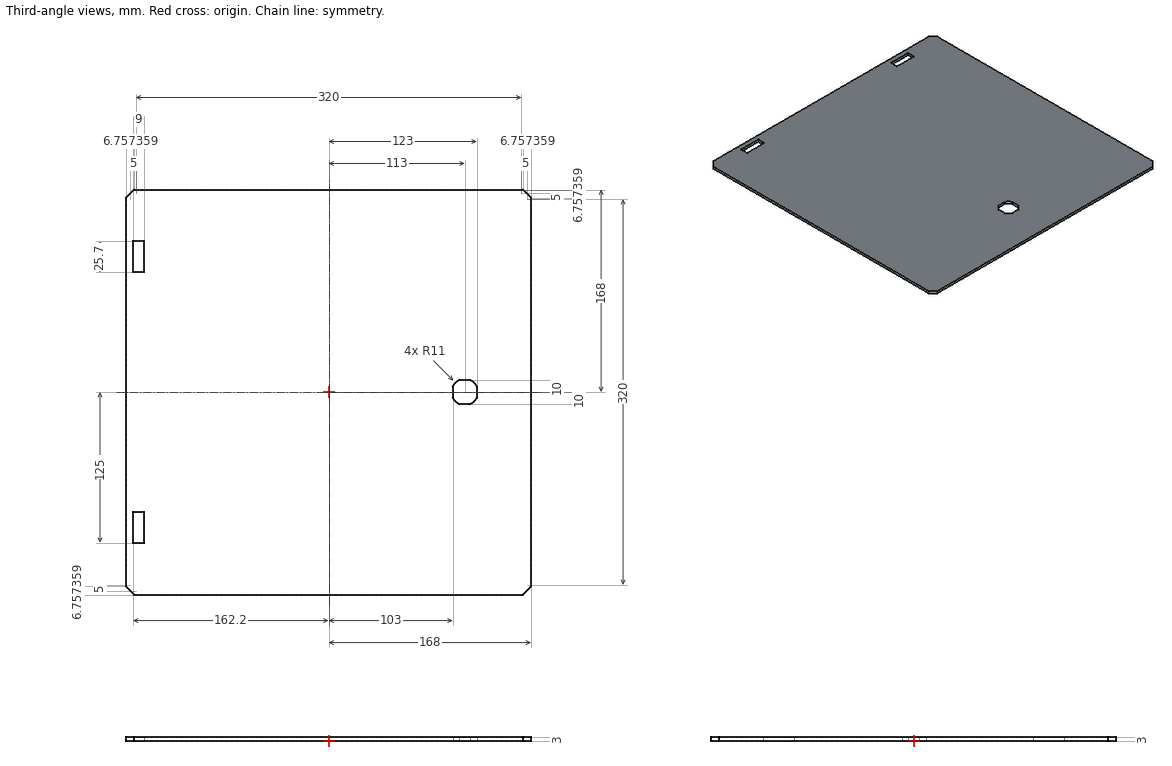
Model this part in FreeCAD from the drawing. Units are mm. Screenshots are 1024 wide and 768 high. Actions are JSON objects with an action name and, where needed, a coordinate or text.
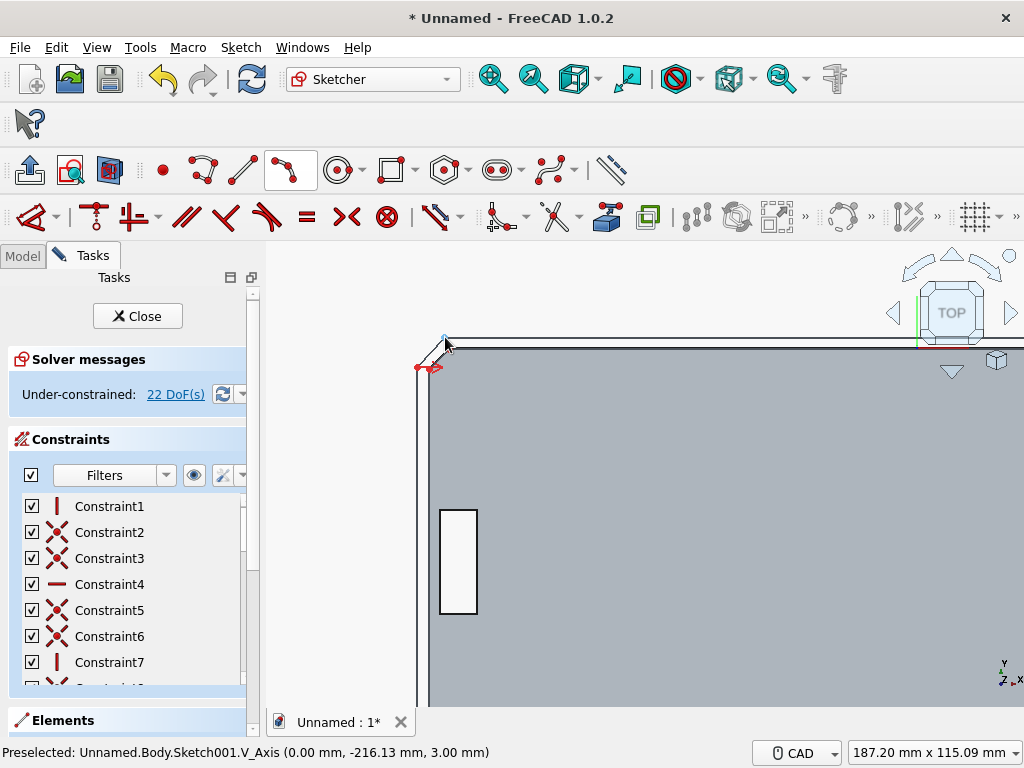
{"action": "left_click", "coordinate": [445, 338]}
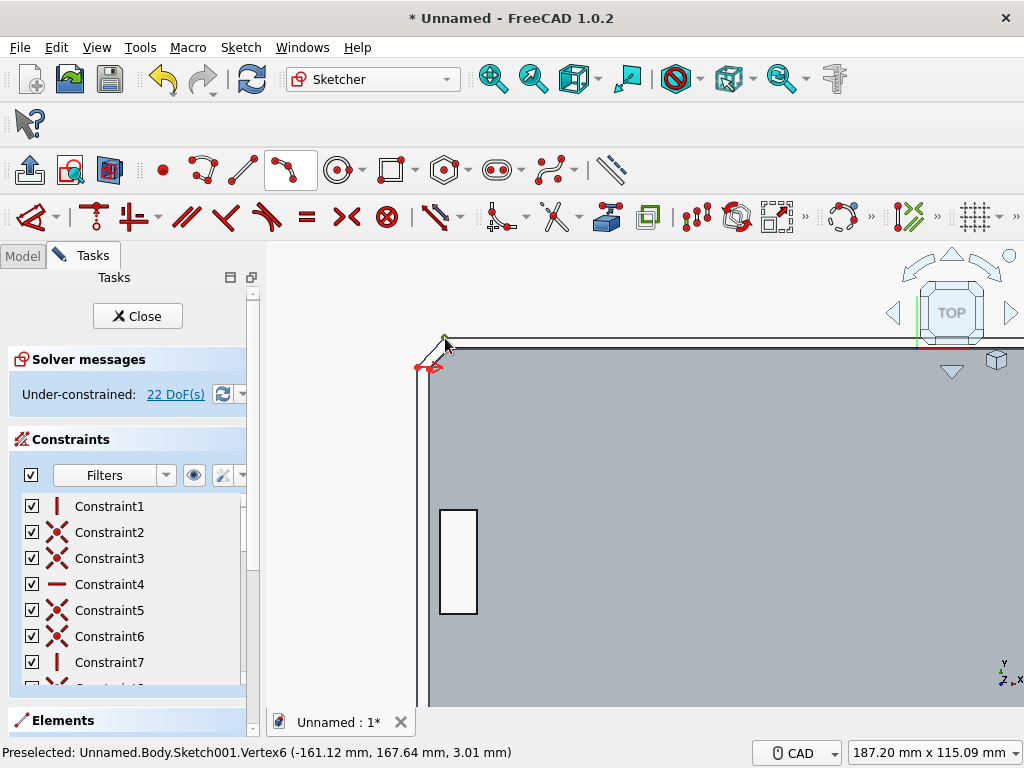
{"action": "scroll", "coordinate": [445, 337], "scroll_direction": "down", "scroll_amount": 8}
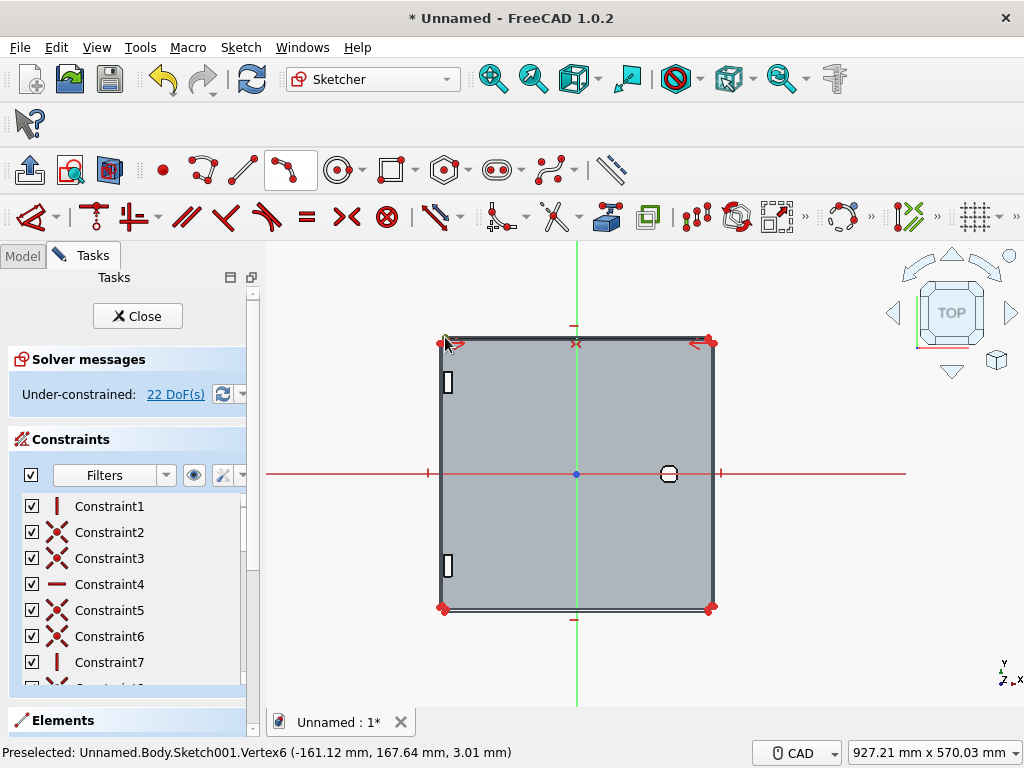
{"action": "scroll", "coordinate": [445, 612], "scroll_direction": "up", "scroll_amount": 7}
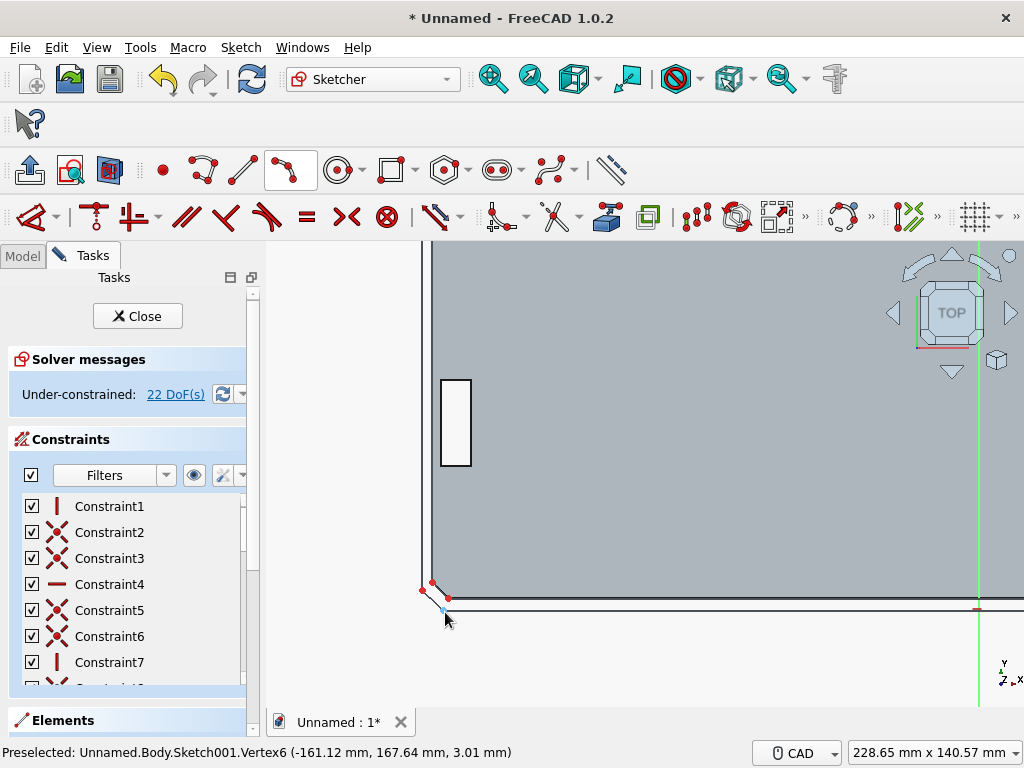
{"action": "left_click", "coordinate": [444, 611]}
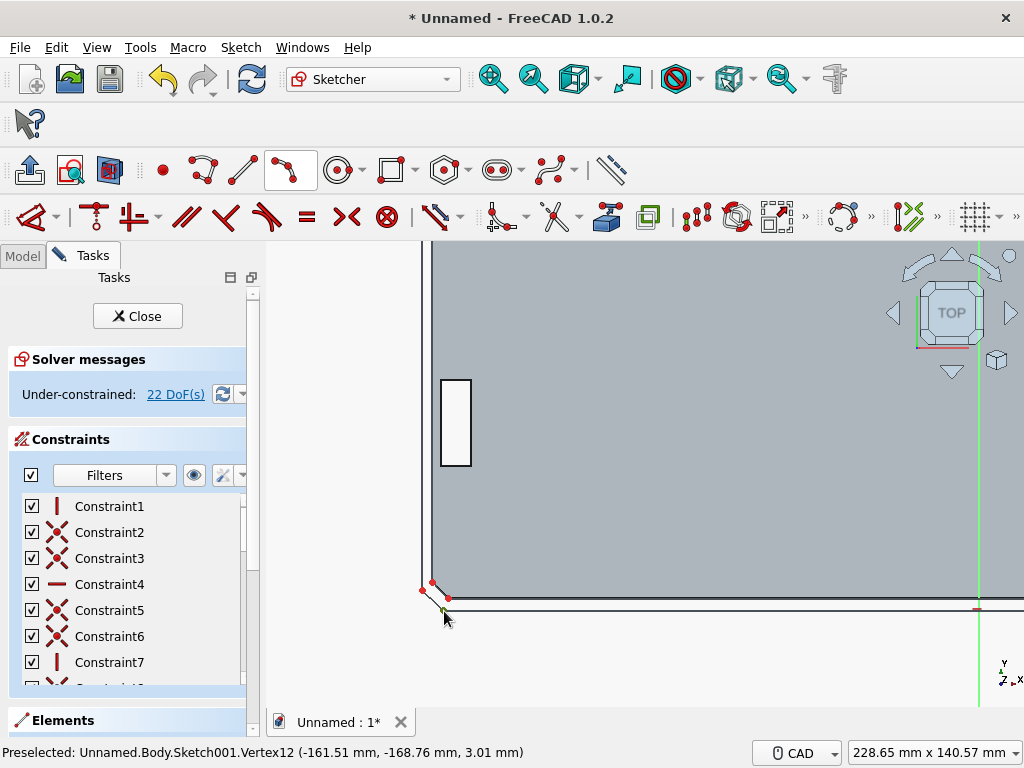
{"action": "scroll", "coordinate": [445, 612], "scroll_direction": "down", "scroll_amount": 7}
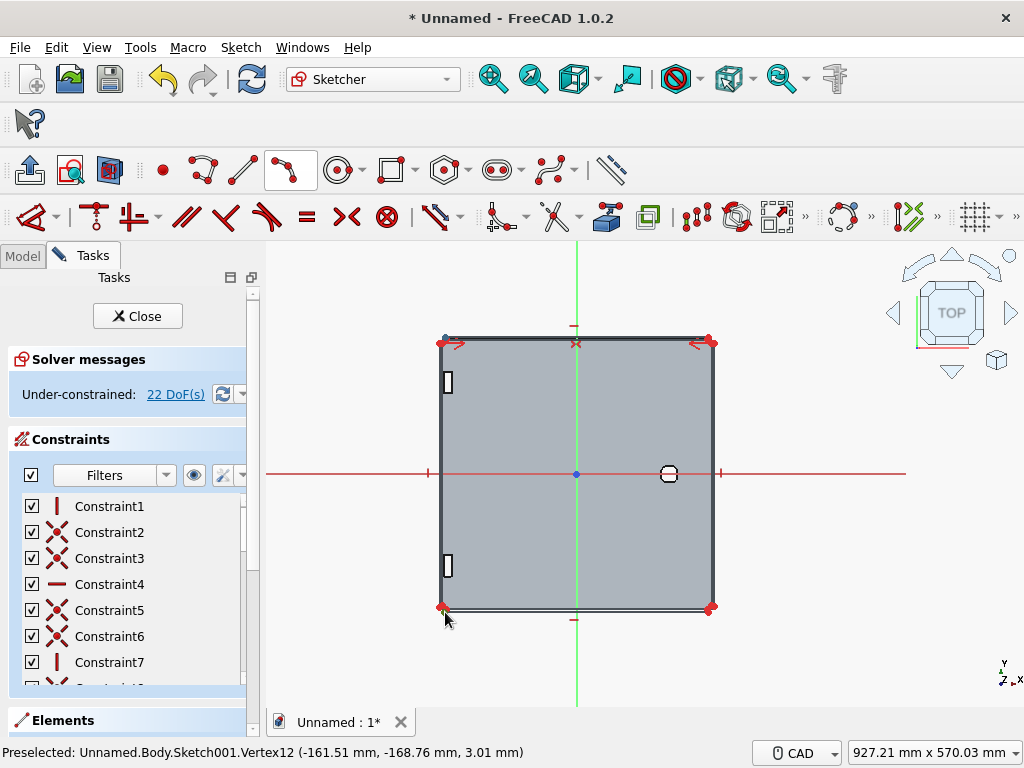
{"action": "left_click", "coordinate": [334, 474]}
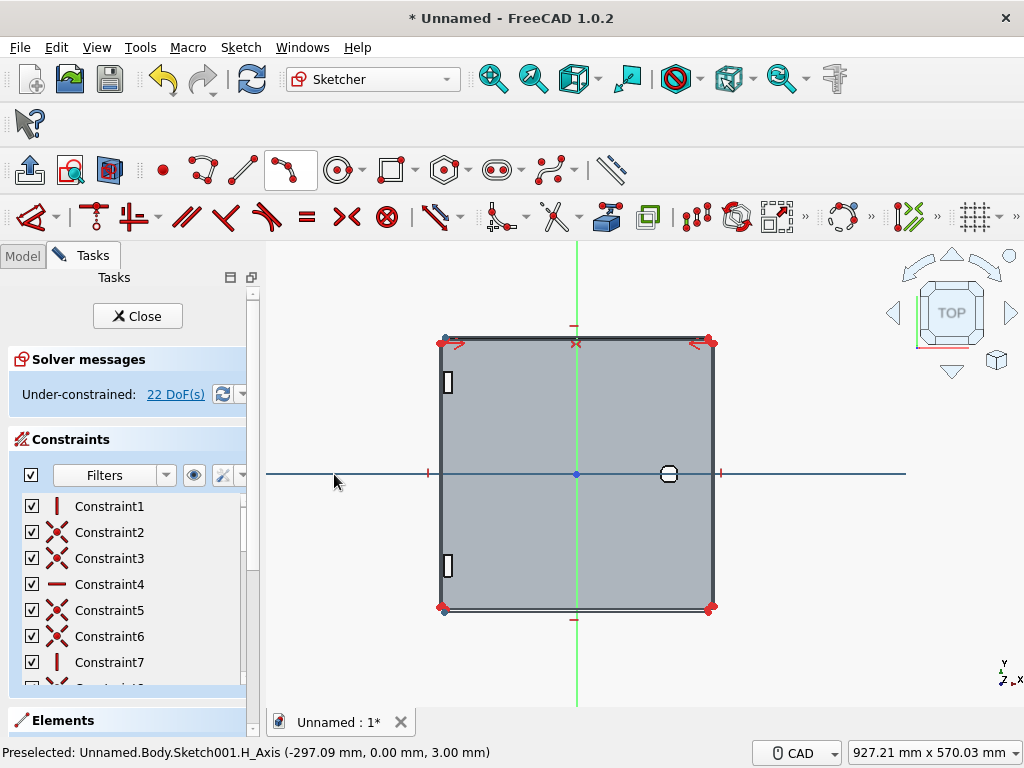
{"action": "left_click", "coordinate": [348, 218]}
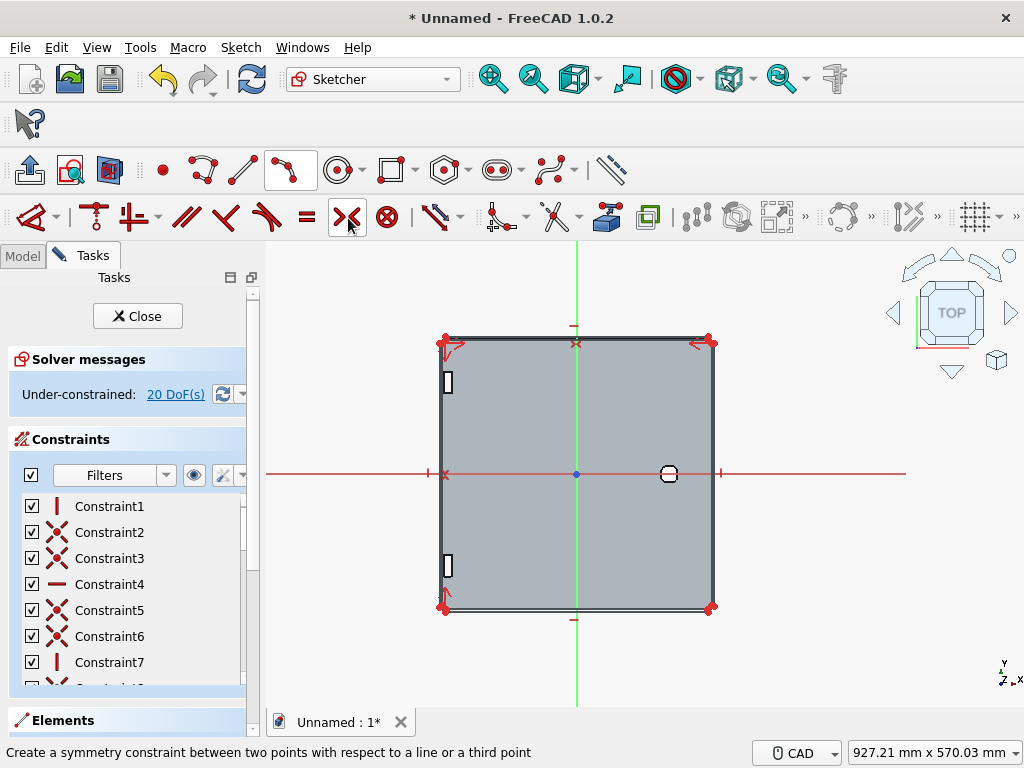
{"action": "scroll", "coordinate": [712, 605], "scroll_direction": "up", "scroll_amount": 8}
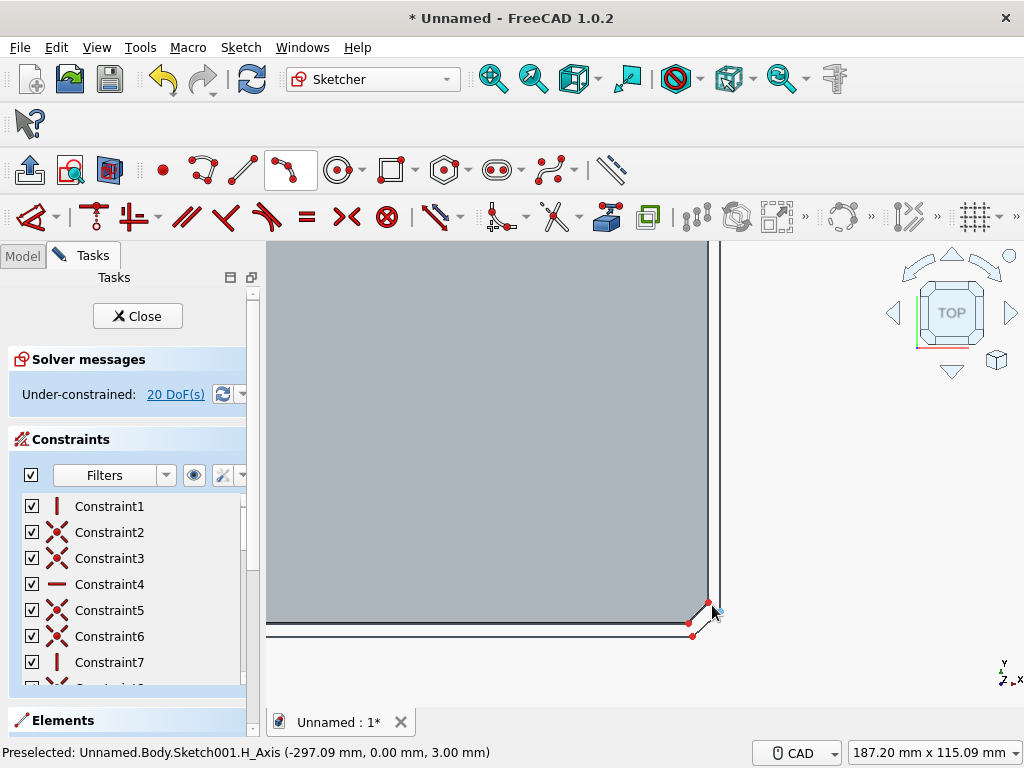
{"action": "left_click", "coordinate": [708, 603]}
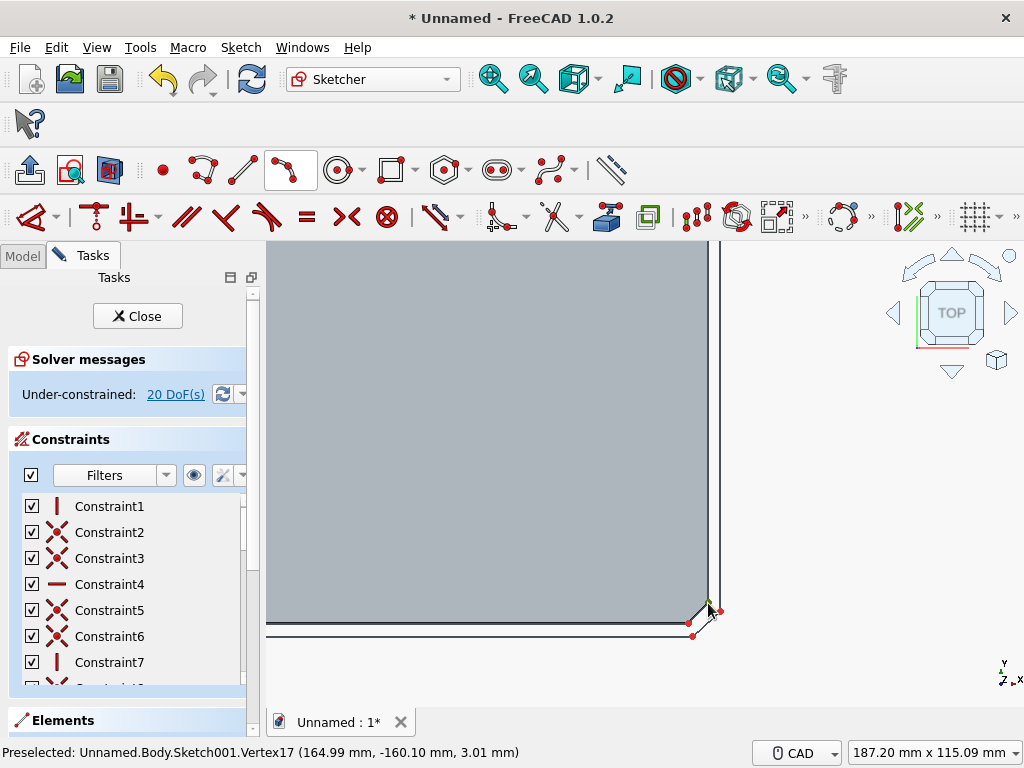
{"action": "scroll", "coordinate": [712, 605], "scroll_direction": "down", "scroll_amount": 8}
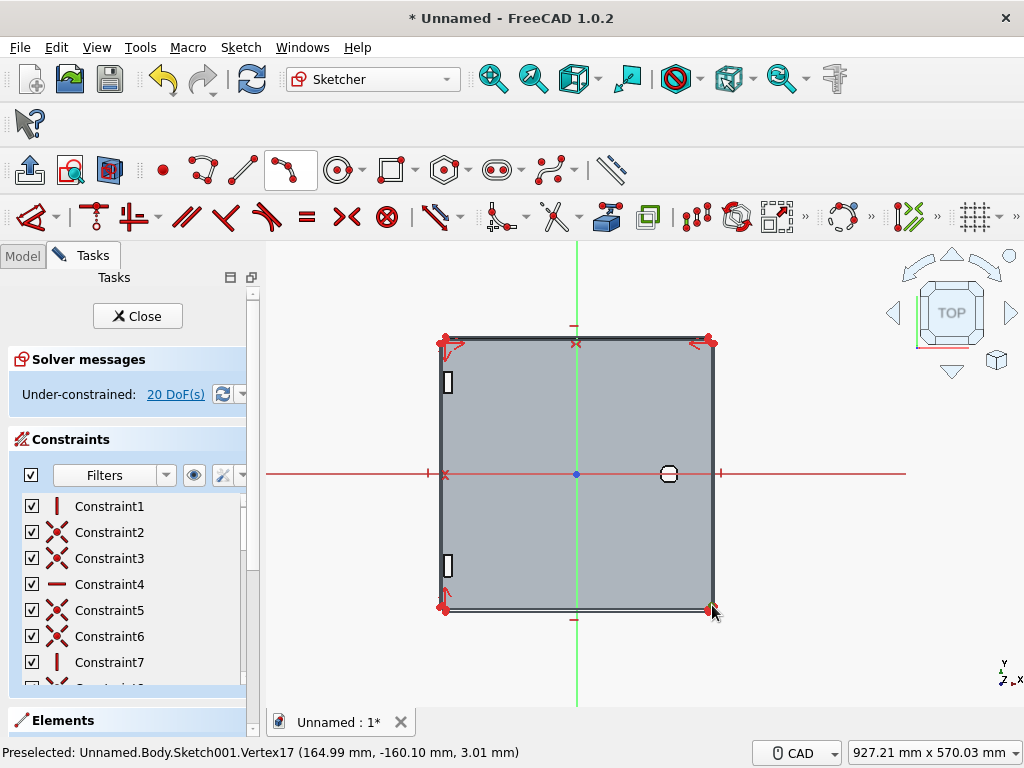
{"action": "scroll", "coordinate": [442, 605], "scroll_direction": "up", "scroll_amount": 7}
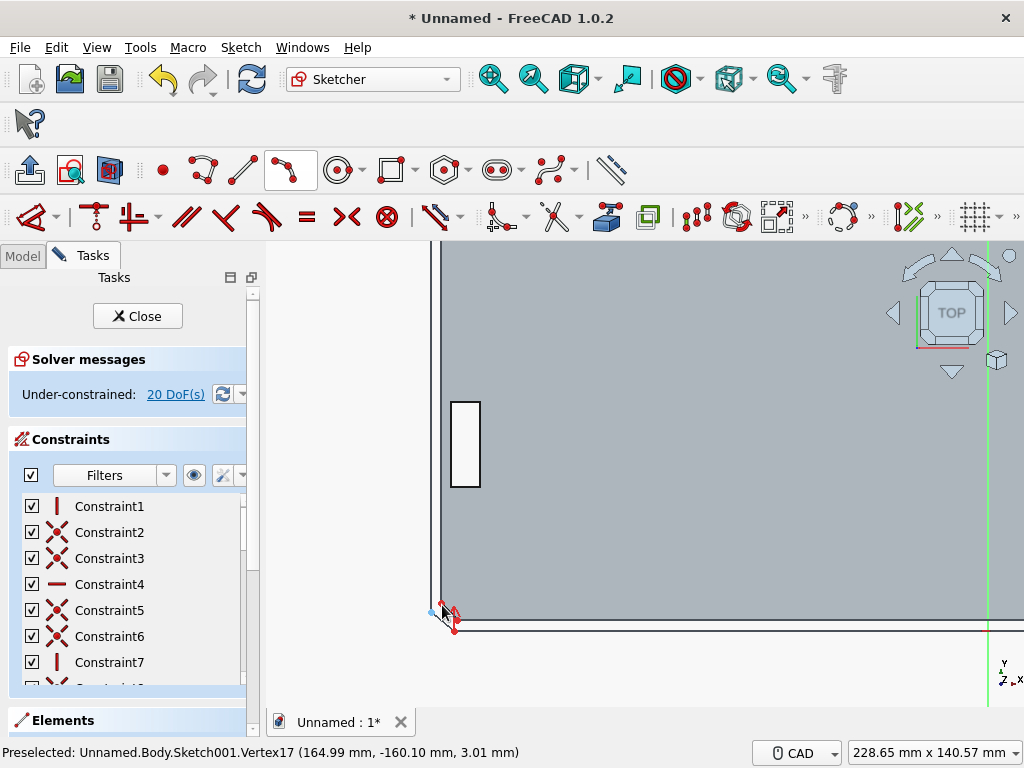
{"action": "left_click", "coordinate": [441, 603]}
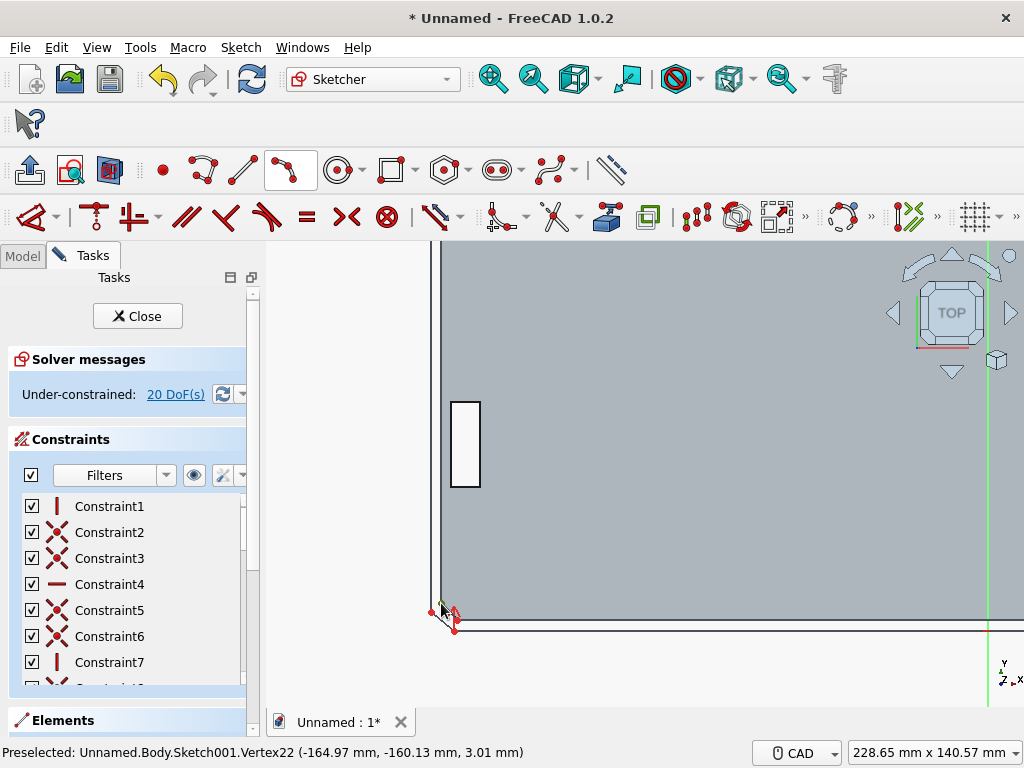
{"action": "scroll", "coordinate": [442, 605], "scroll_direction": "down", "scroll_amount": 7}